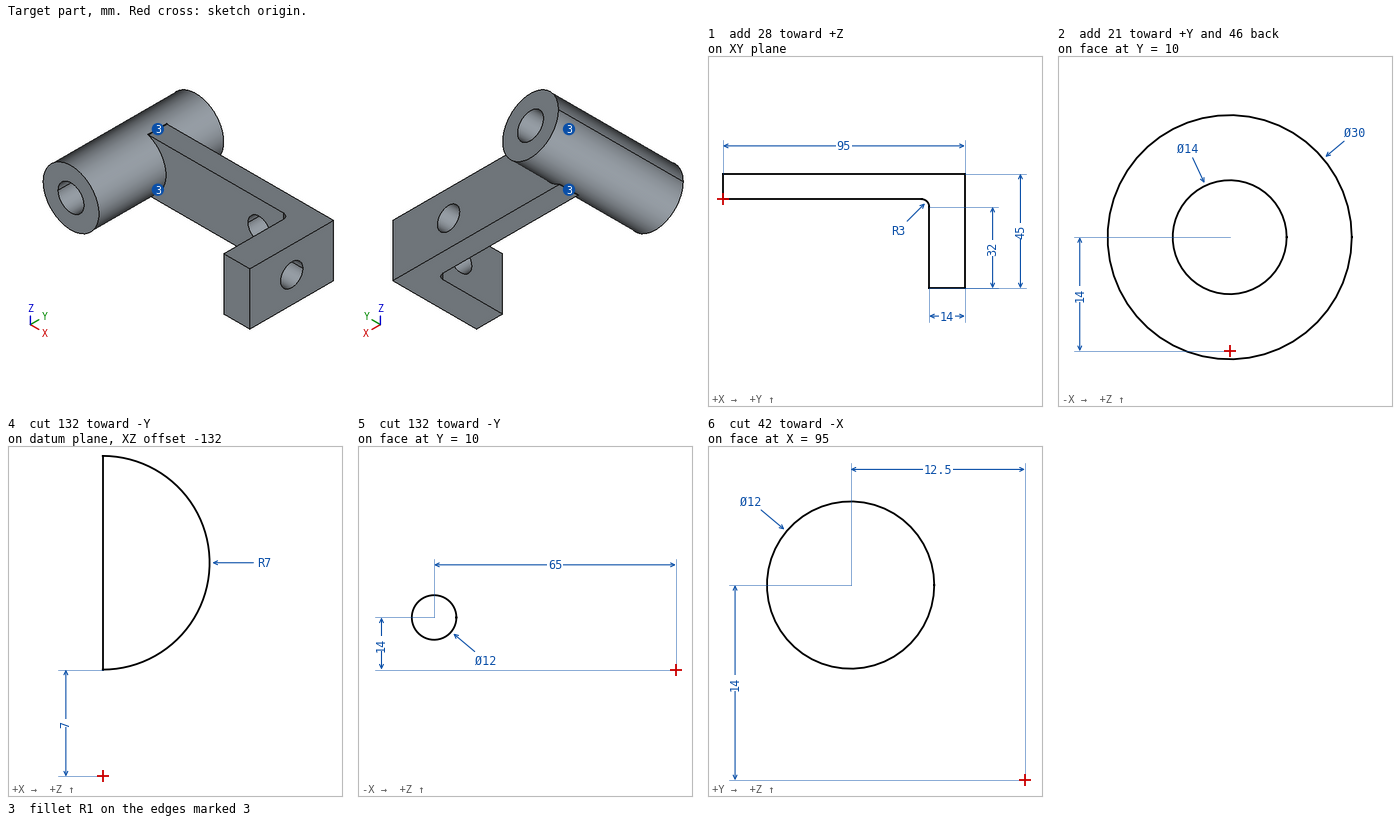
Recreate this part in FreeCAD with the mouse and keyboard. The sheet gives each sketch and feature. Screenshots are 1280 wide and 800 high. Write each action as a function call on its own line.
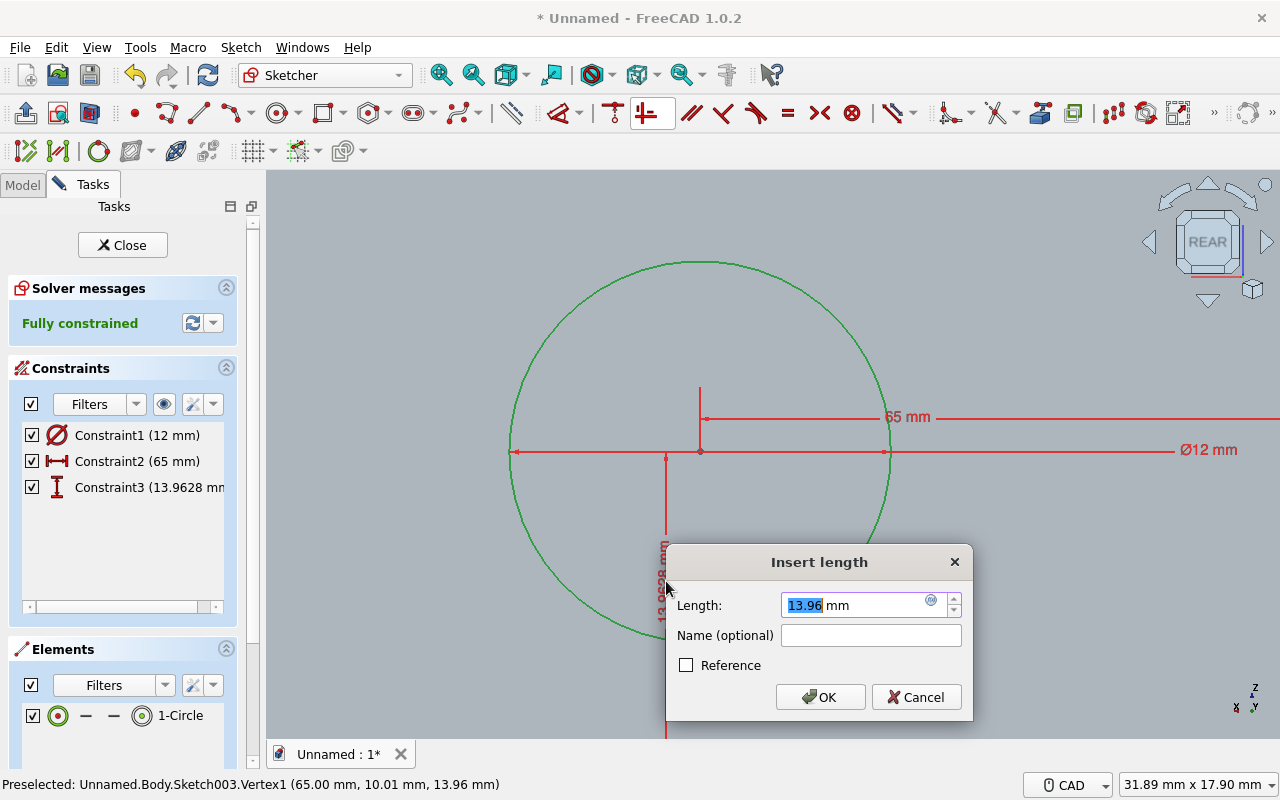
text(14)
key(Return)
key(Escape)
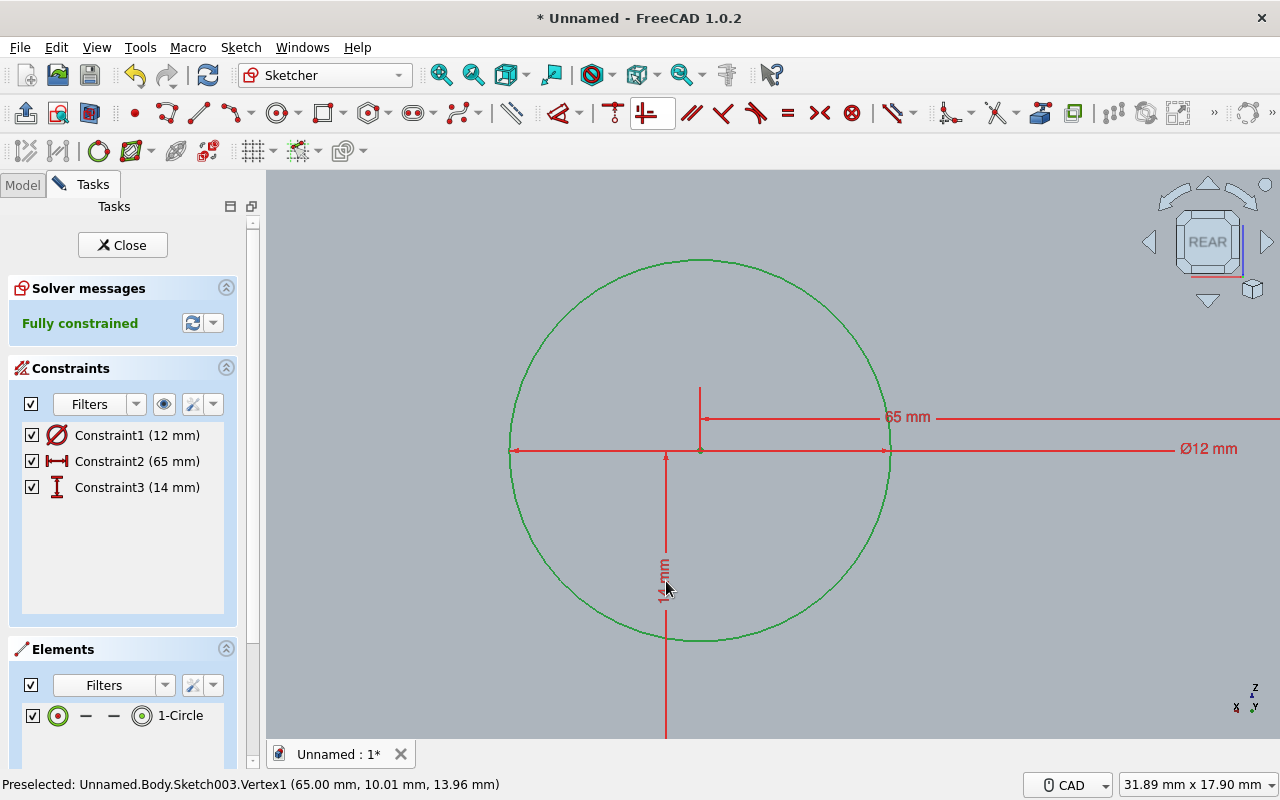
click(123, 245)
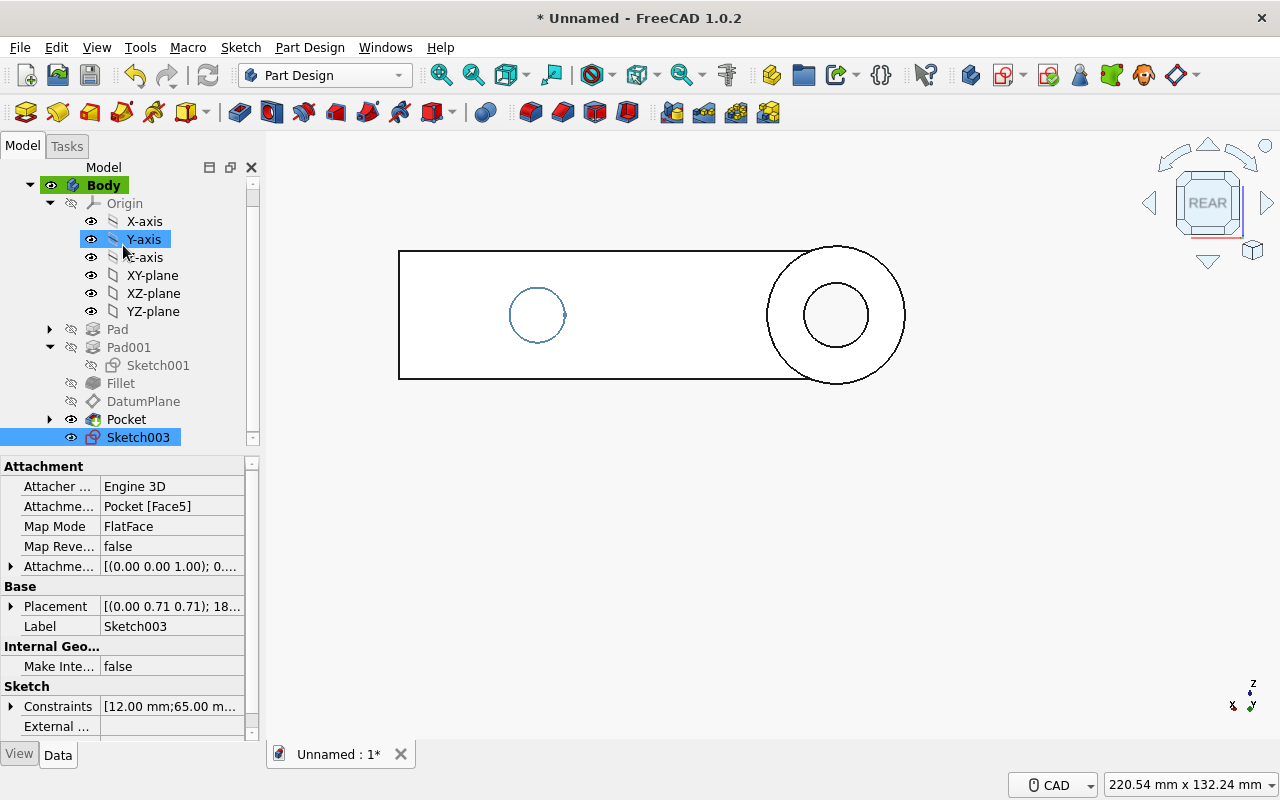
click(240, 112)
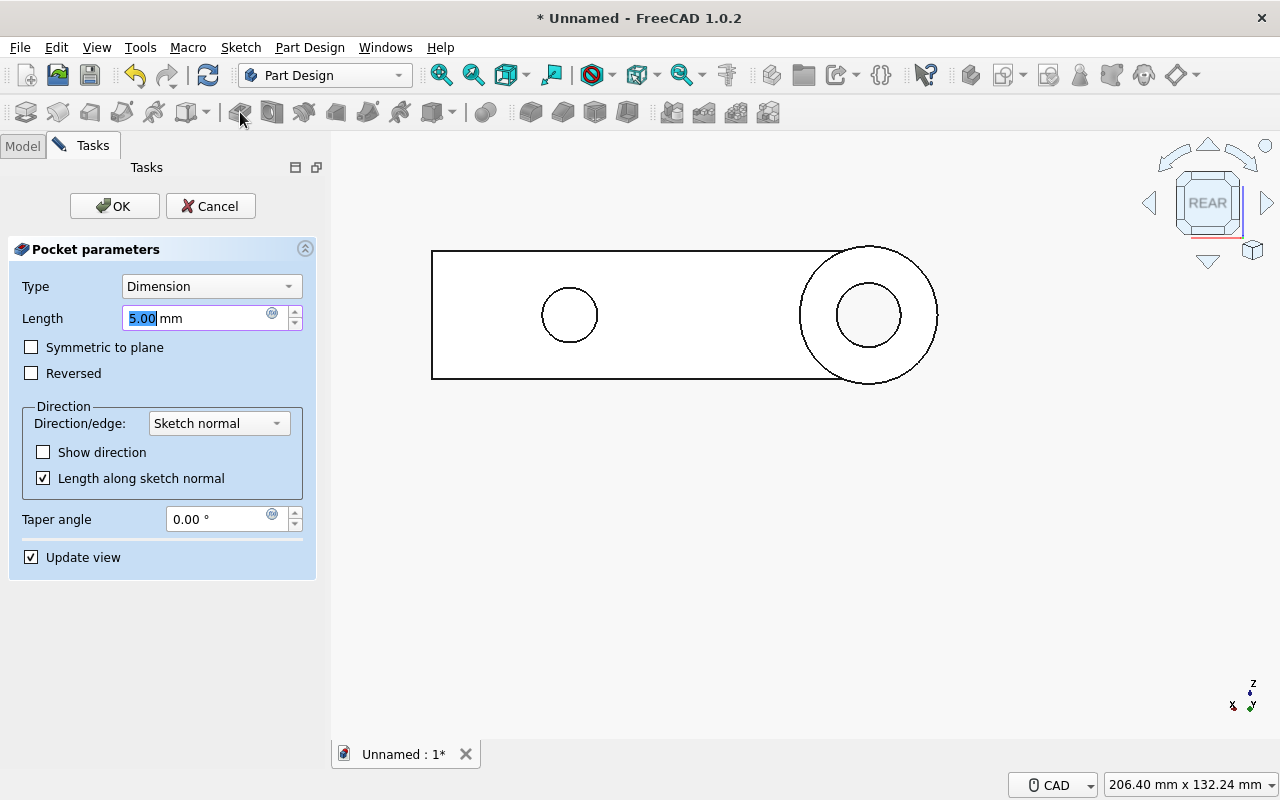
text(132)
key(Tab)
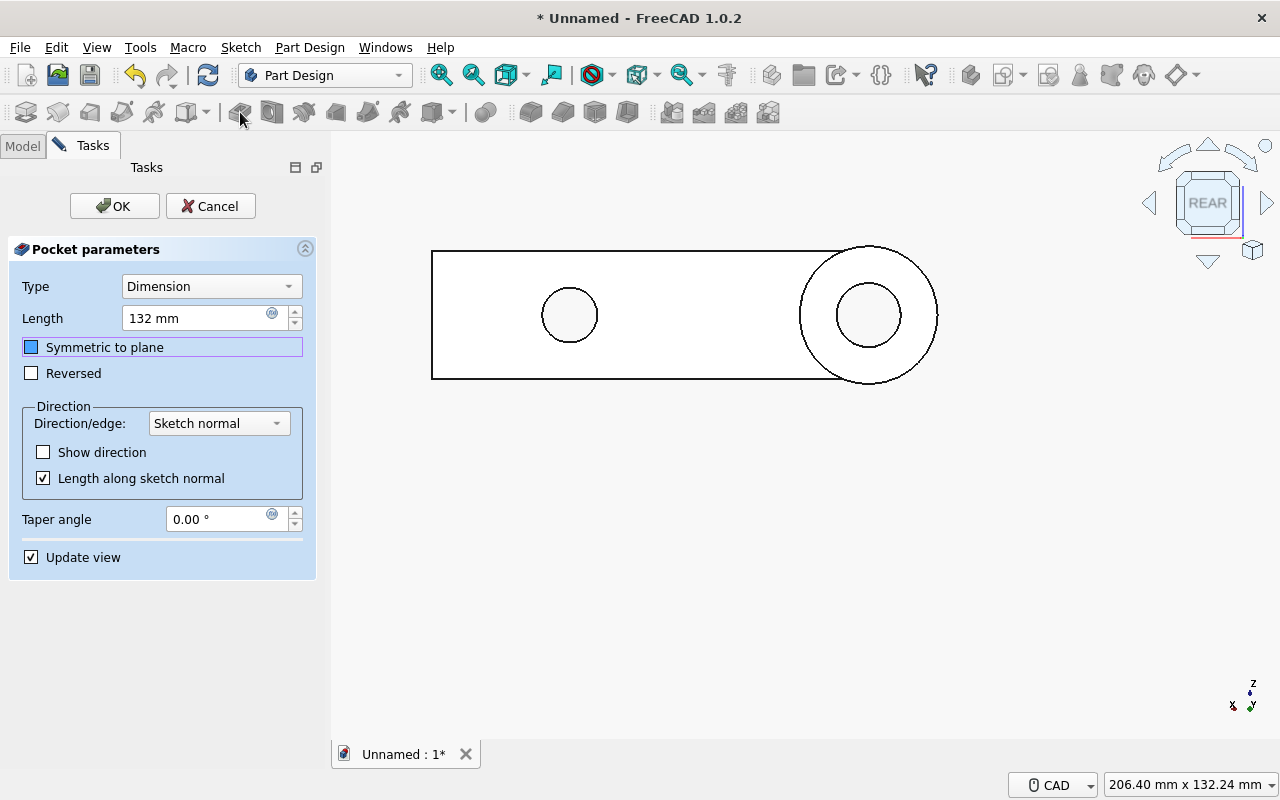
click(115, 206)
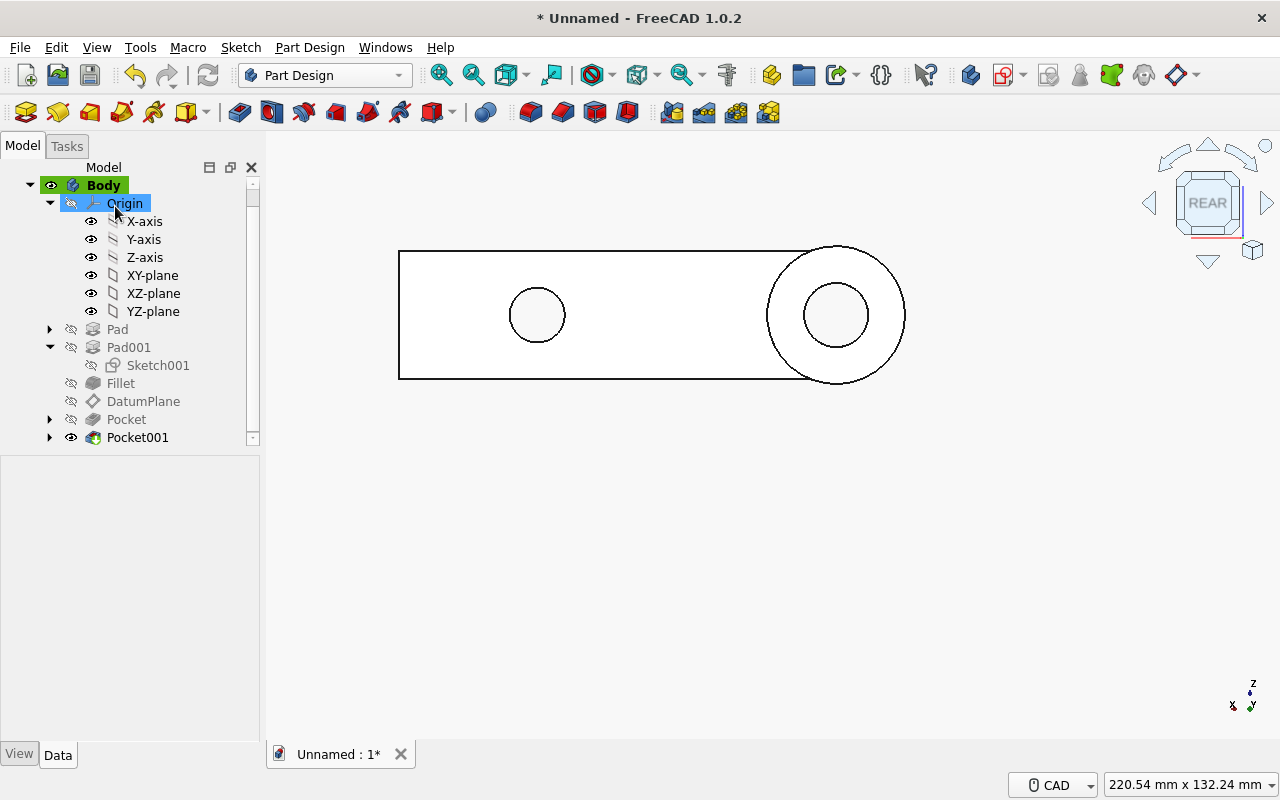
key(0)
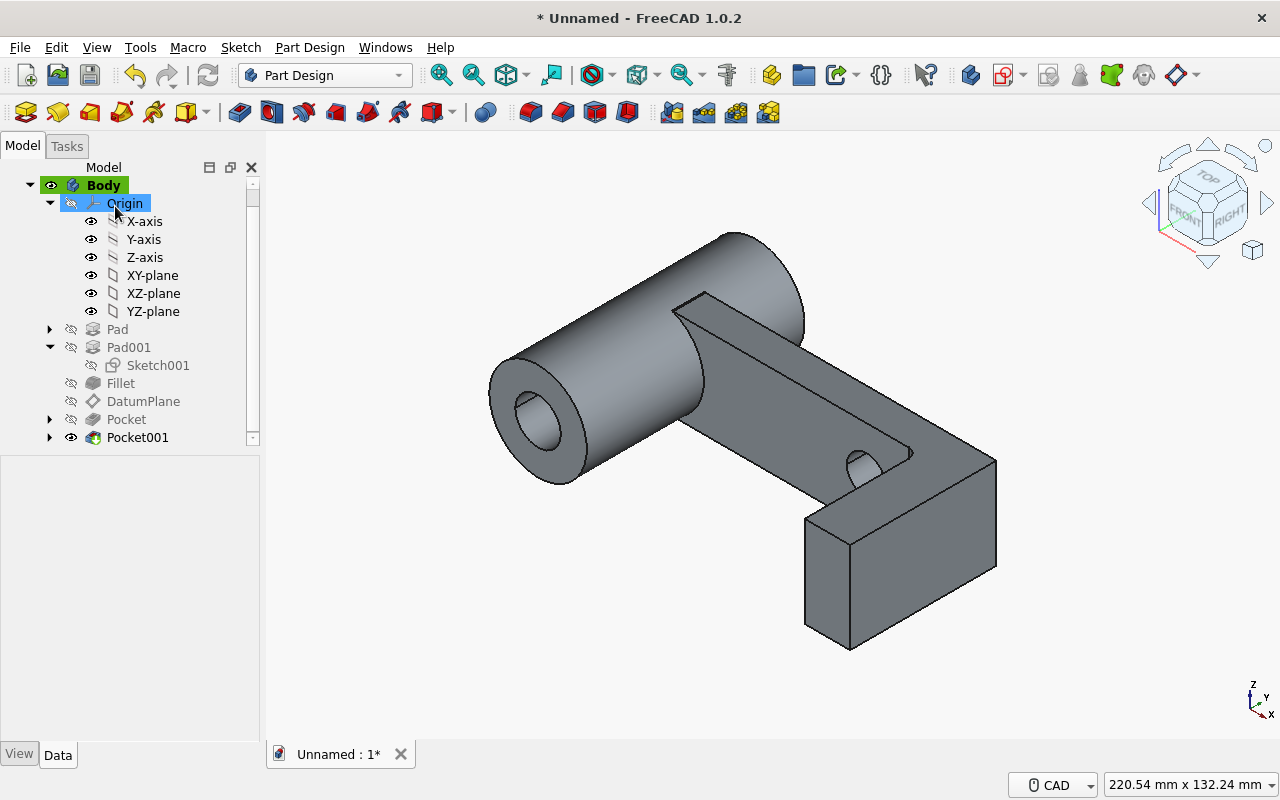
click(944, 542)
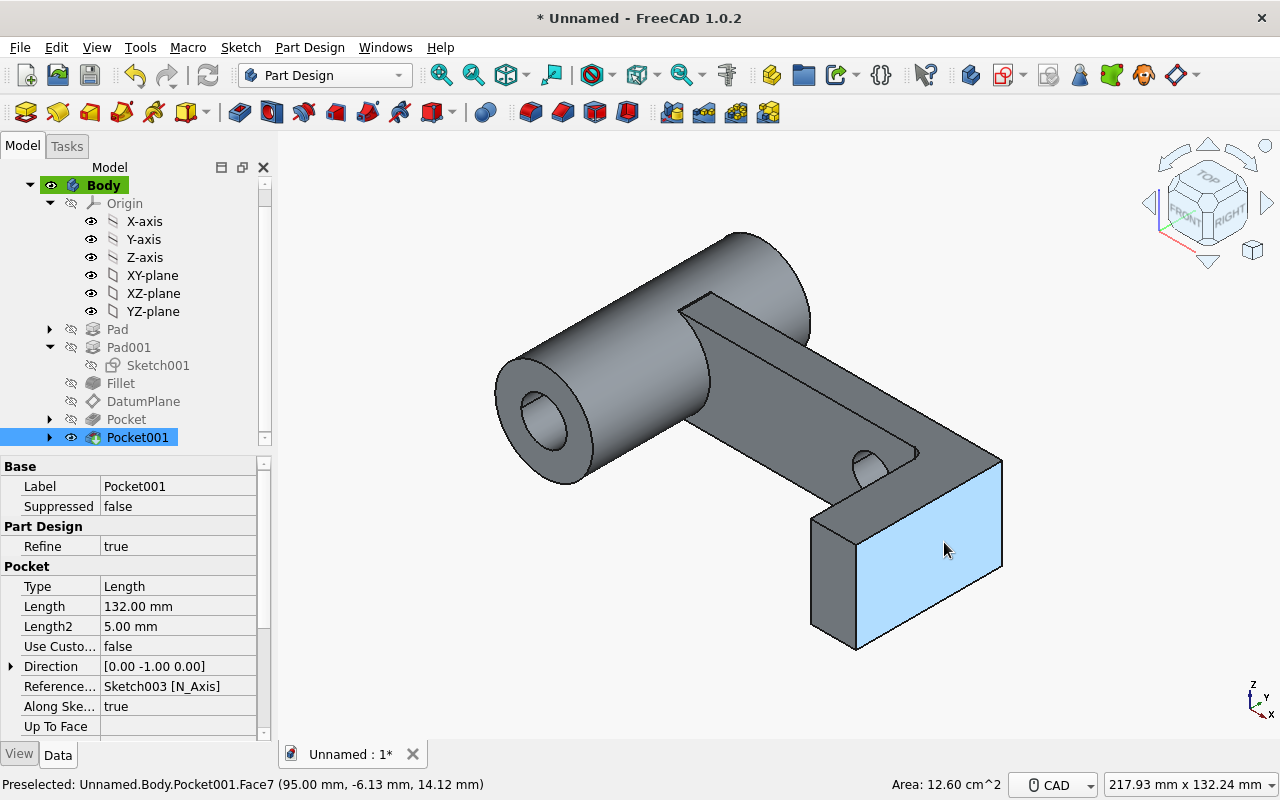
click(1004, 76)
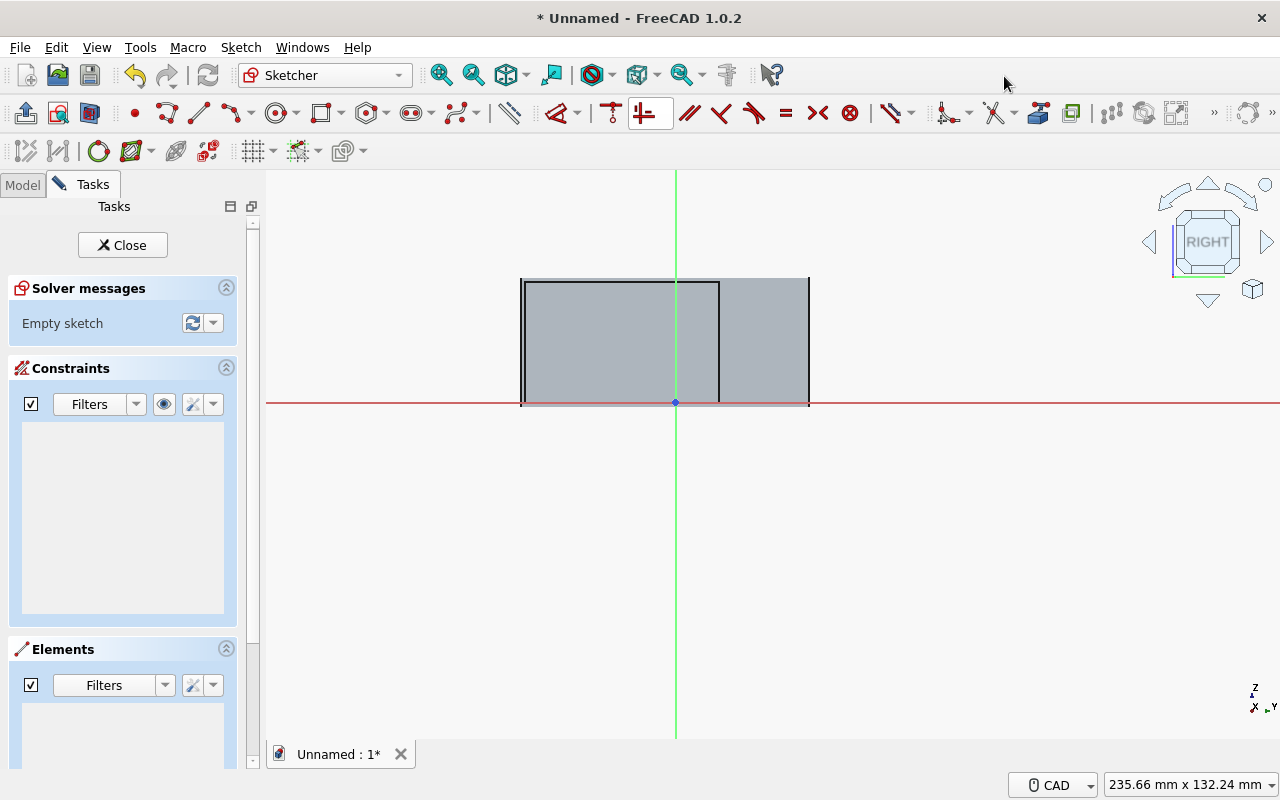
scroll(614, 328, up, 7)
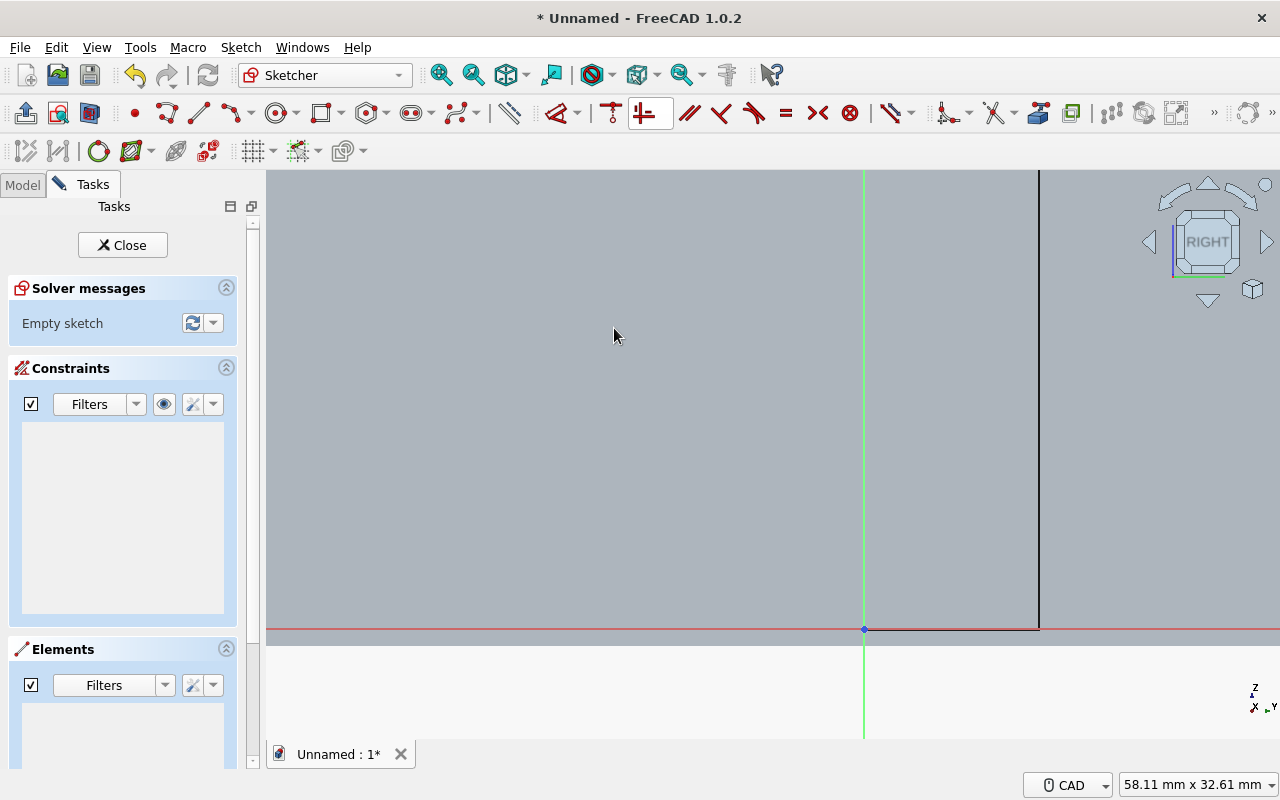
click(276, 114)